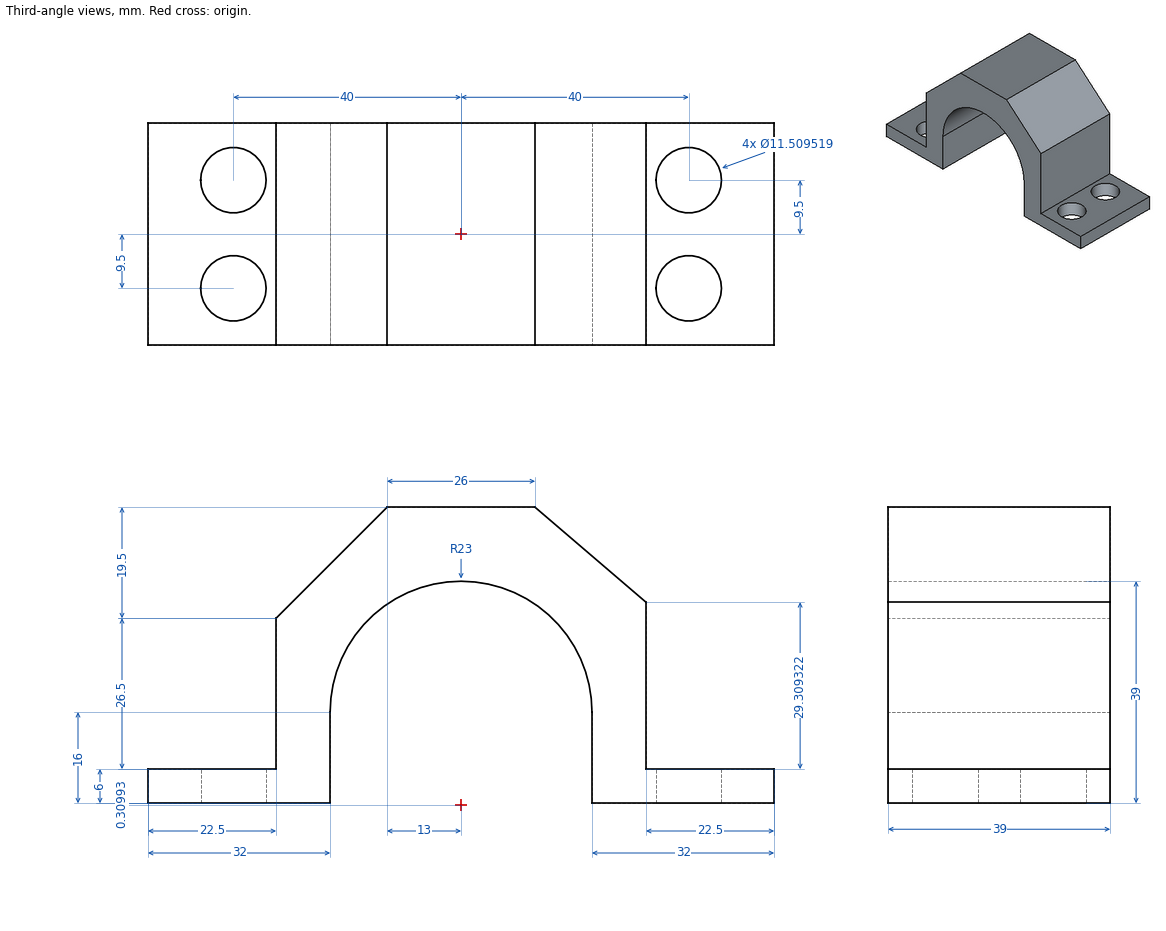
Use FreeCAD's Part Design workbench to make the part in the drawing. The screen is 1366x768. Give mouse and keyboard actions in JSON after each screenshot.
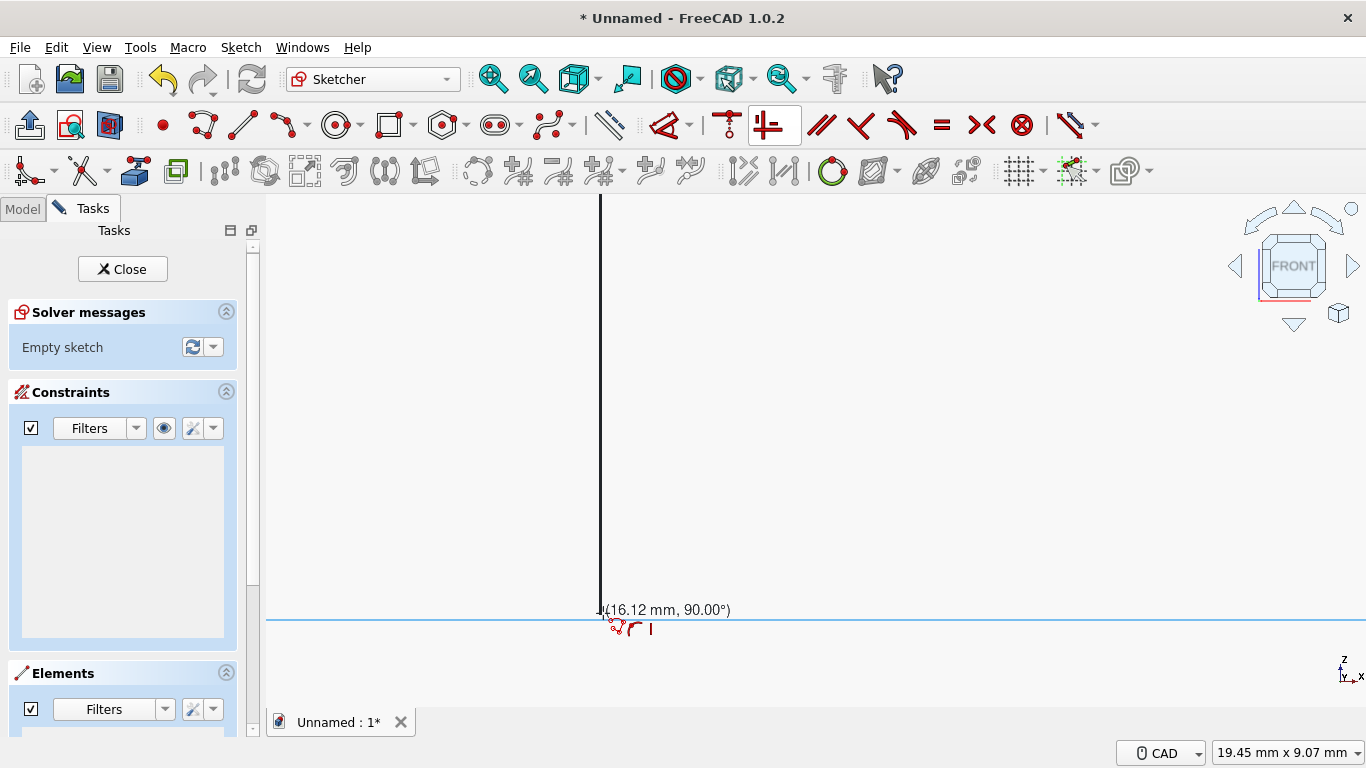
{"action": "left_click", "coordinate": [601, 603]}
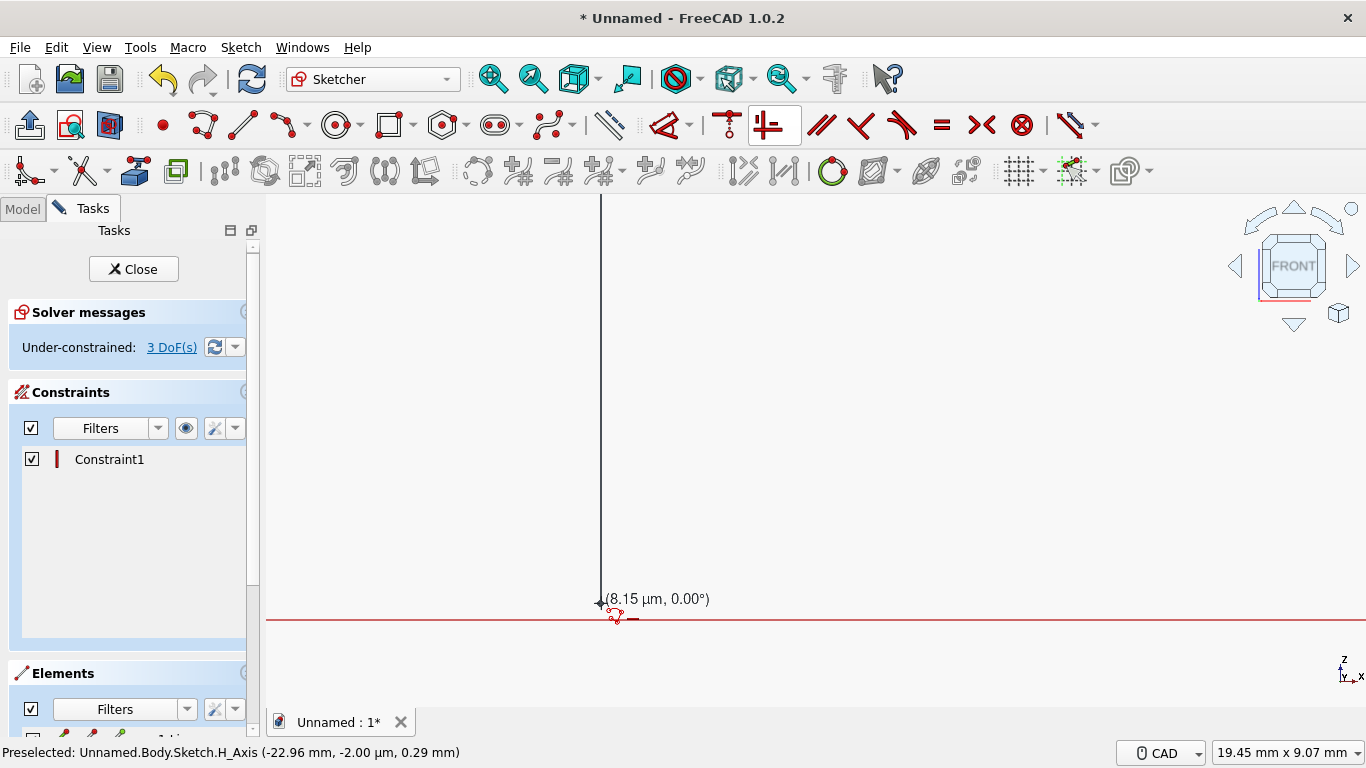
{"action": "scroll", "coordinate": [604, 614], "scroll_direction": "down", "scroll_amount": 11}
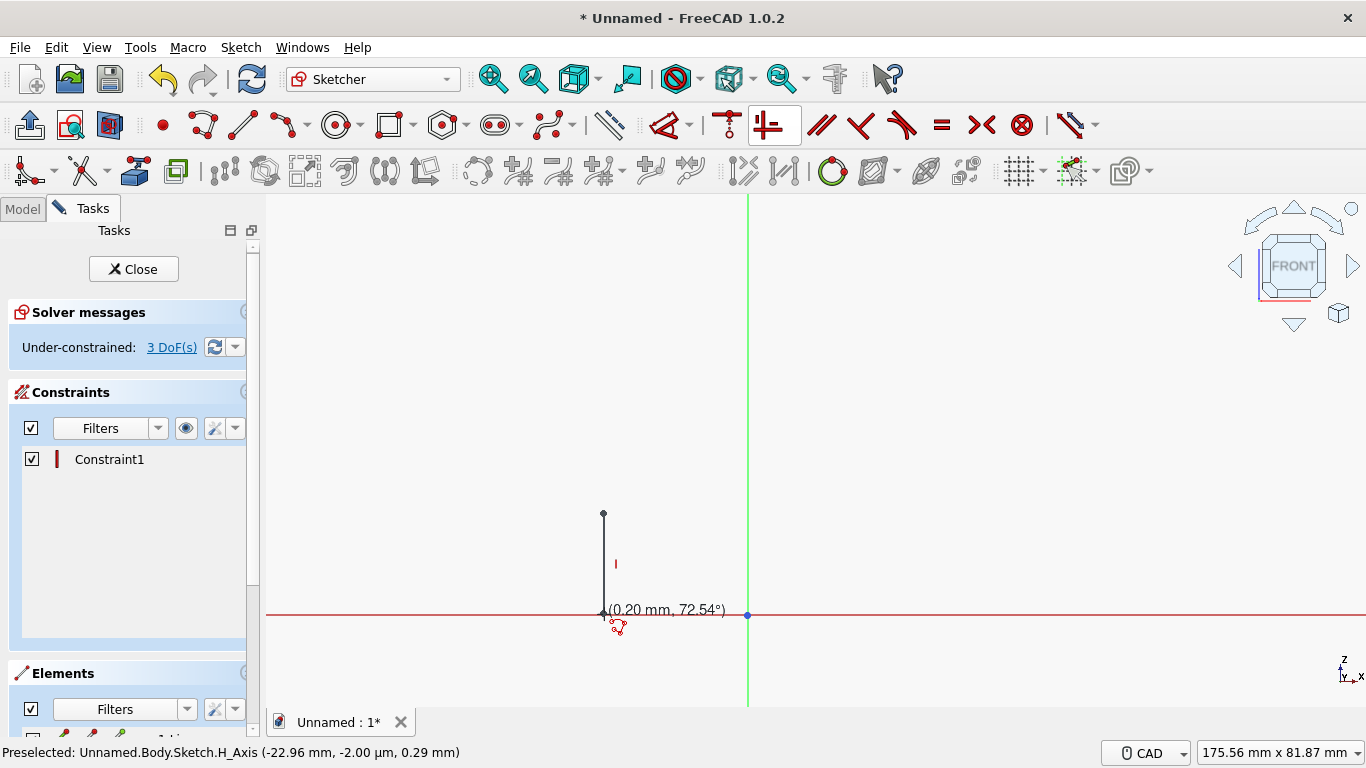
{"action": "scroll", "coordinate": [403, 614], "scroll_direction": "up", "scroll_amount": 11}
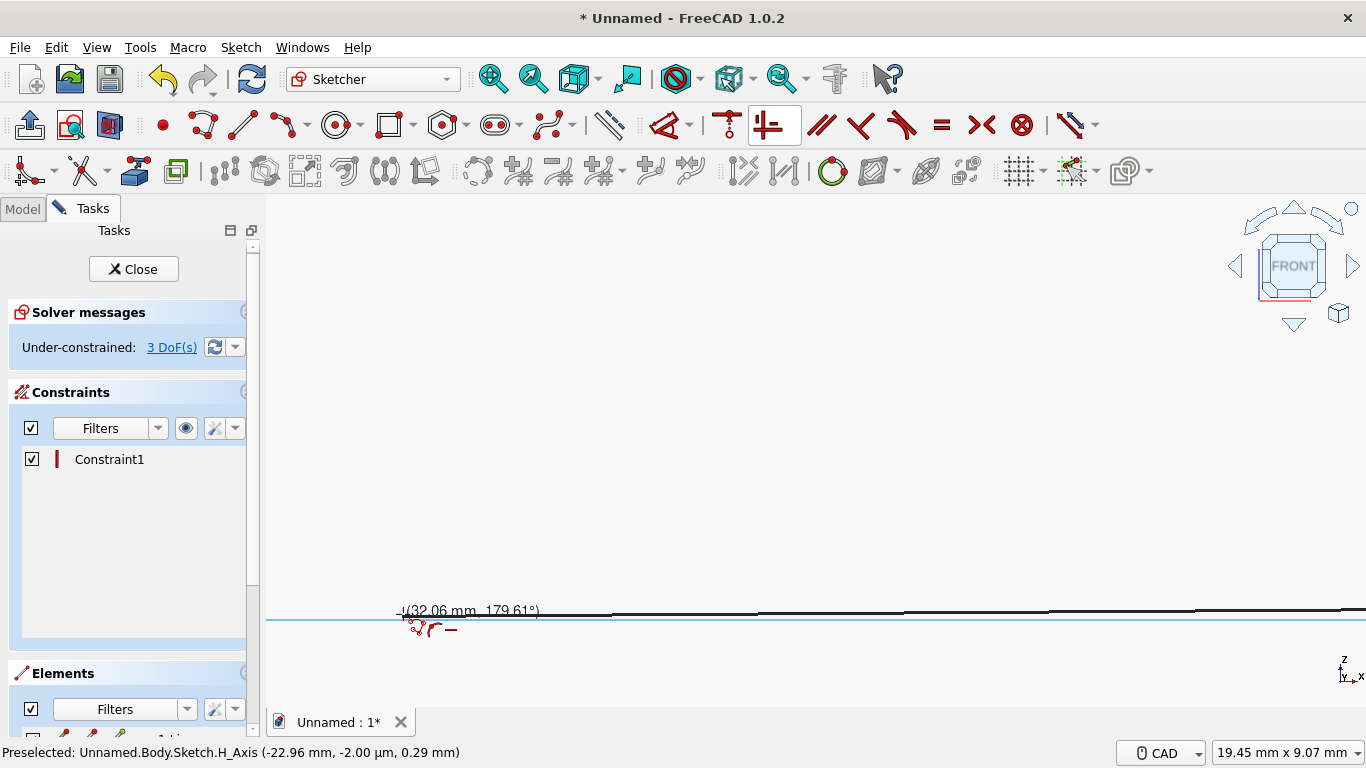
{"action": "left_click", "coordinate": [405, 603]}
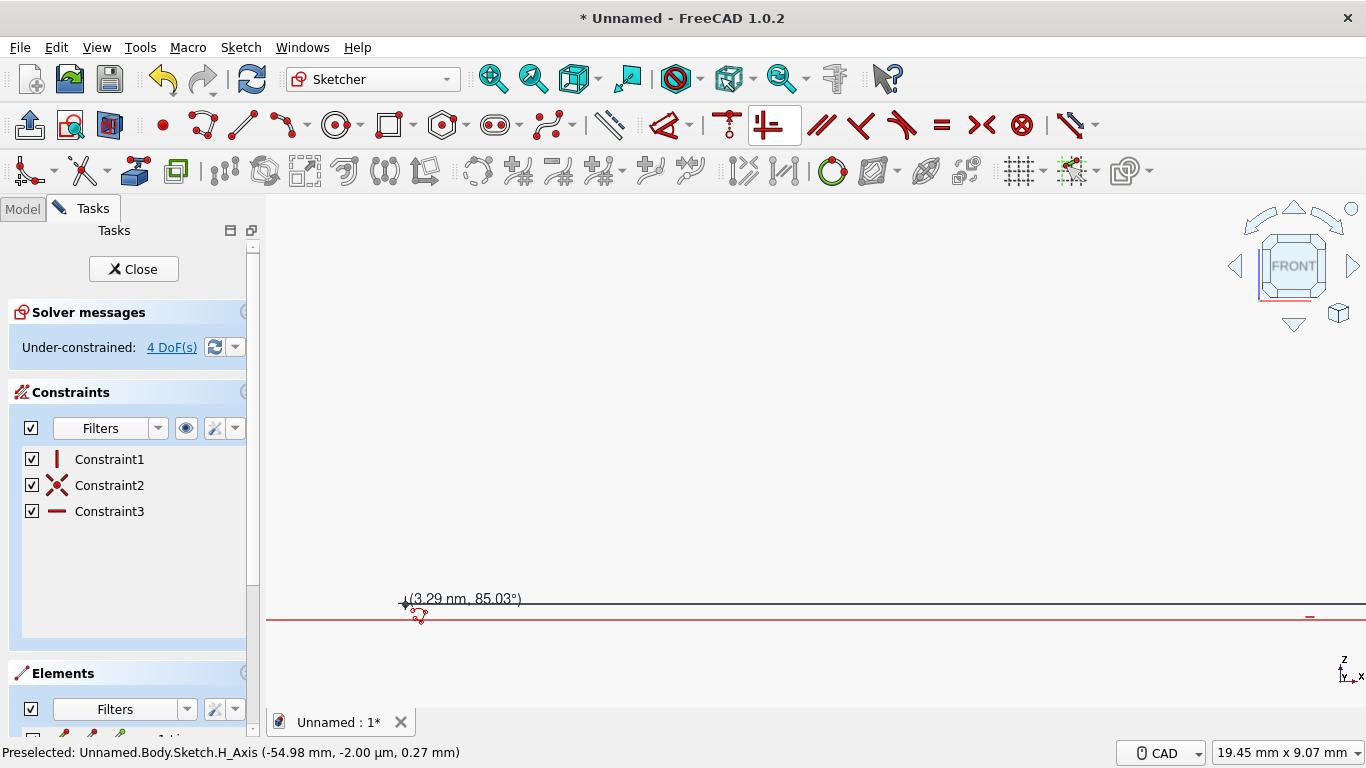
{"action": "scroll", "coordinate": [403, 614], "scroll_direction": "down", "scroll_amount": 11}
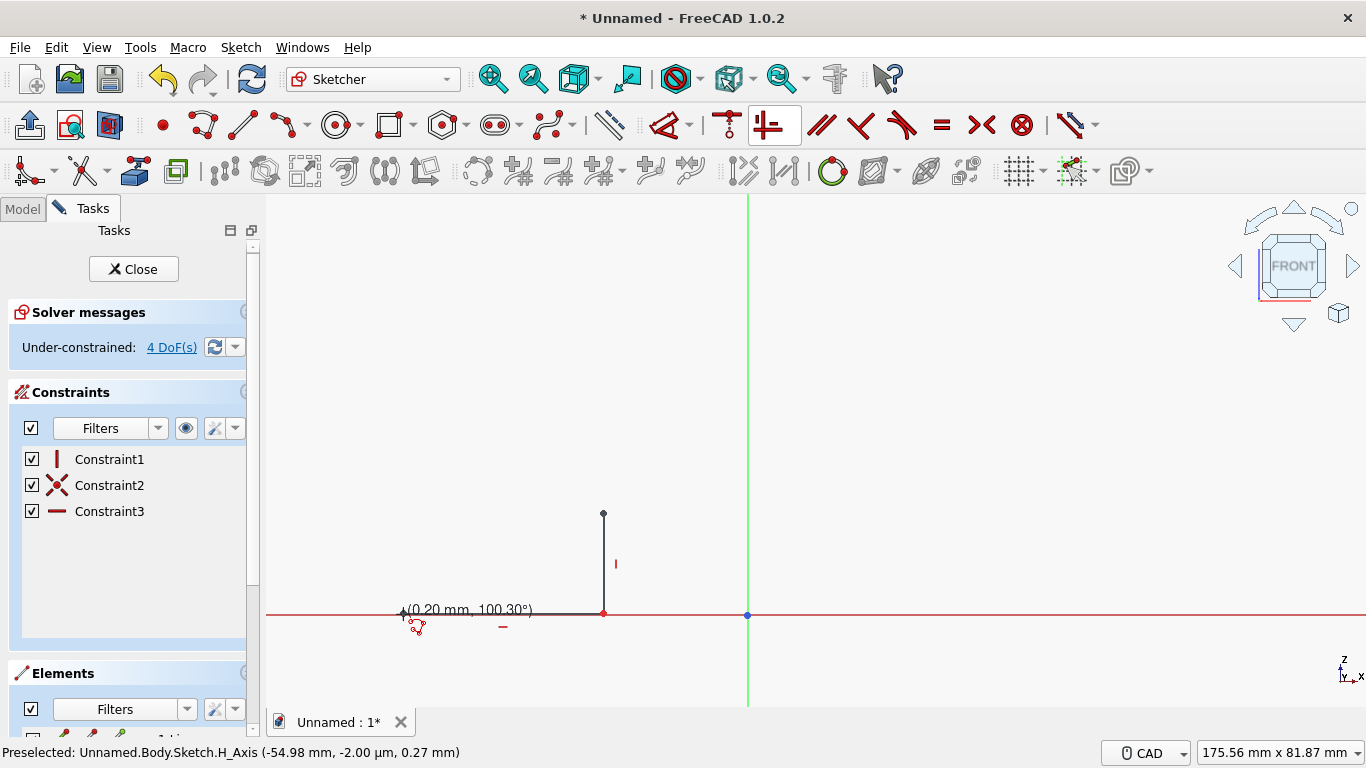
{"action": "left_click", "coordinate": [403, 576]}
{"action": "left_click", "coordinate": [544, 576]}
{"action": "left_click", "coordinate": [544, 410]}
{"action": "left_click", "coordinate": [666, 288]}
{"action": "left_click", "coordinate": [829, 288]}
{"action": "left_click", "coordinate": [952, 392]}
{"action": "left_click", "coordinate": [952, 576]}
{"action": "left_click", "coordinate": [1093, 576]}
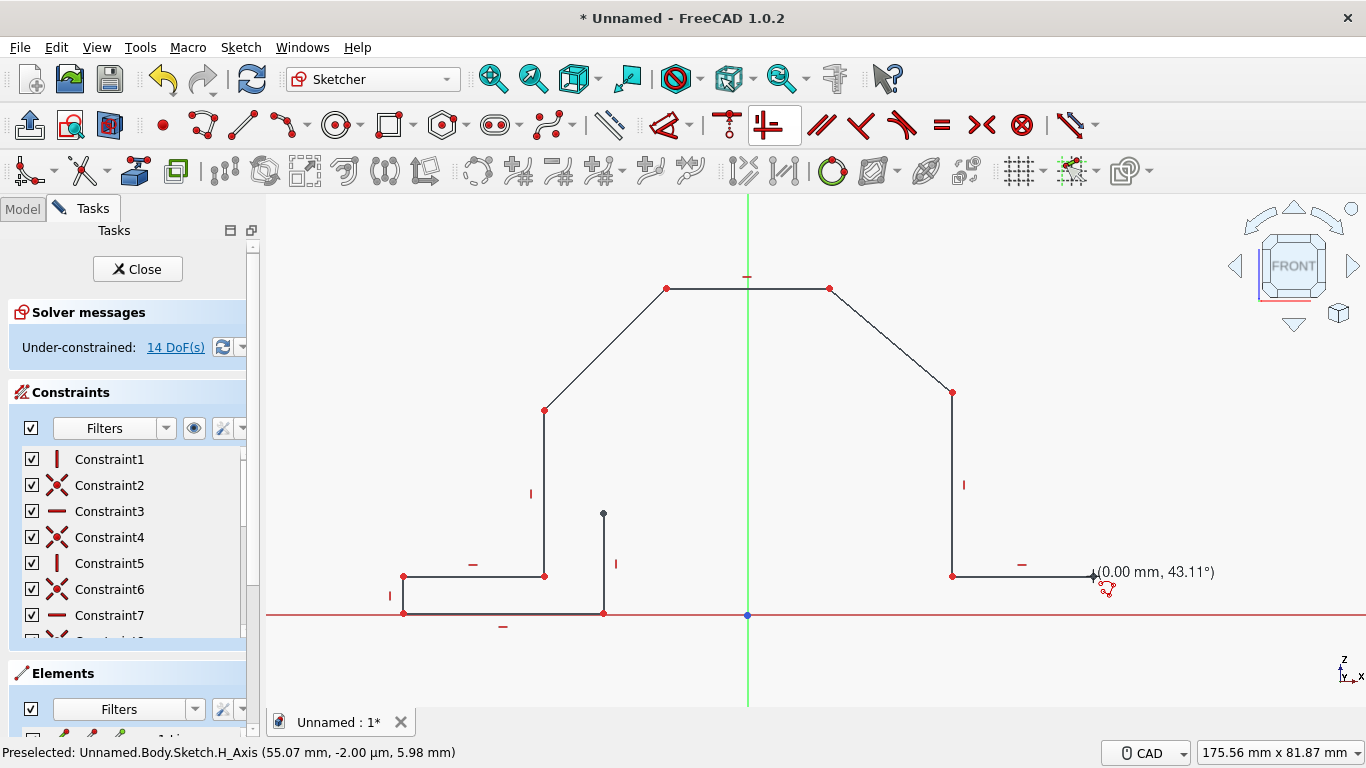
{"action": "scroll", "coordinate": [1093, 614], "scroll_direction": "up", "scroll_amount": 11}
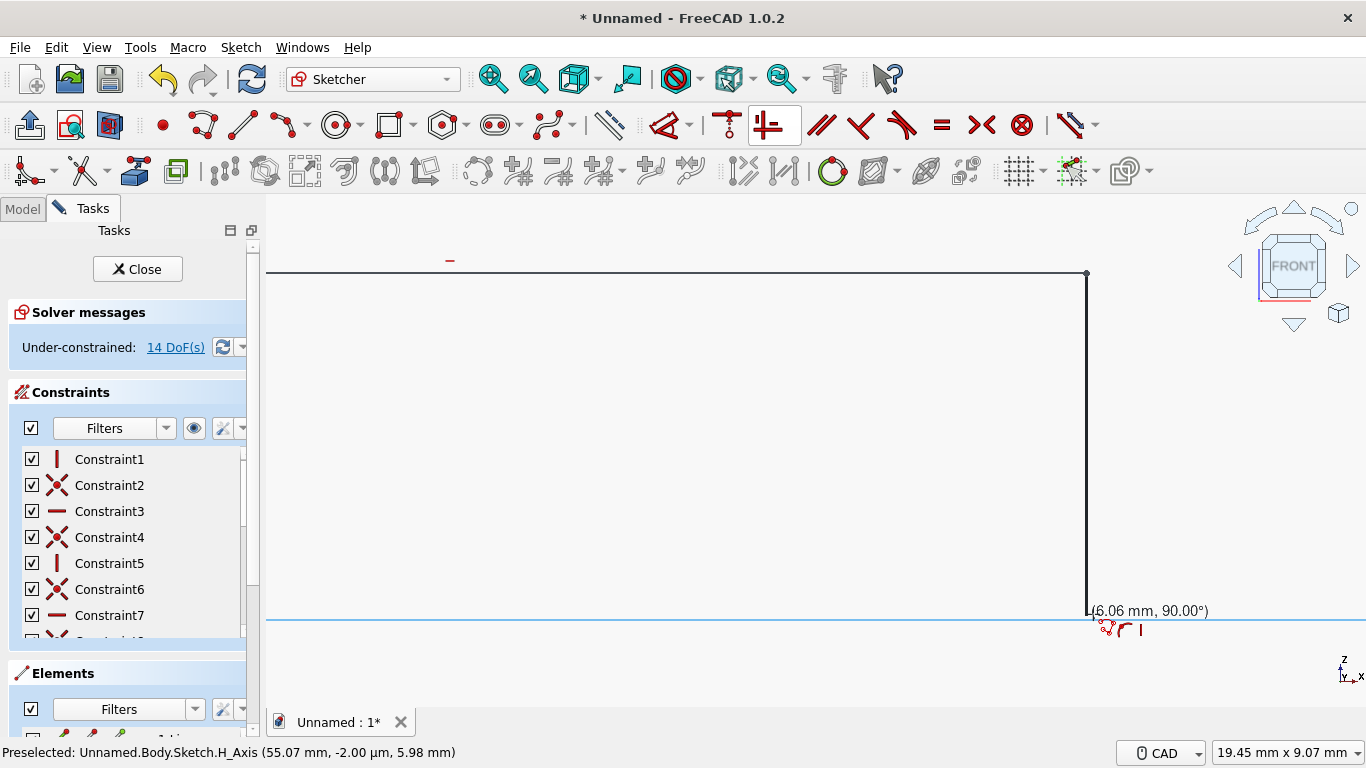
{"action": "left_click", "coordinate": [1087, 603]}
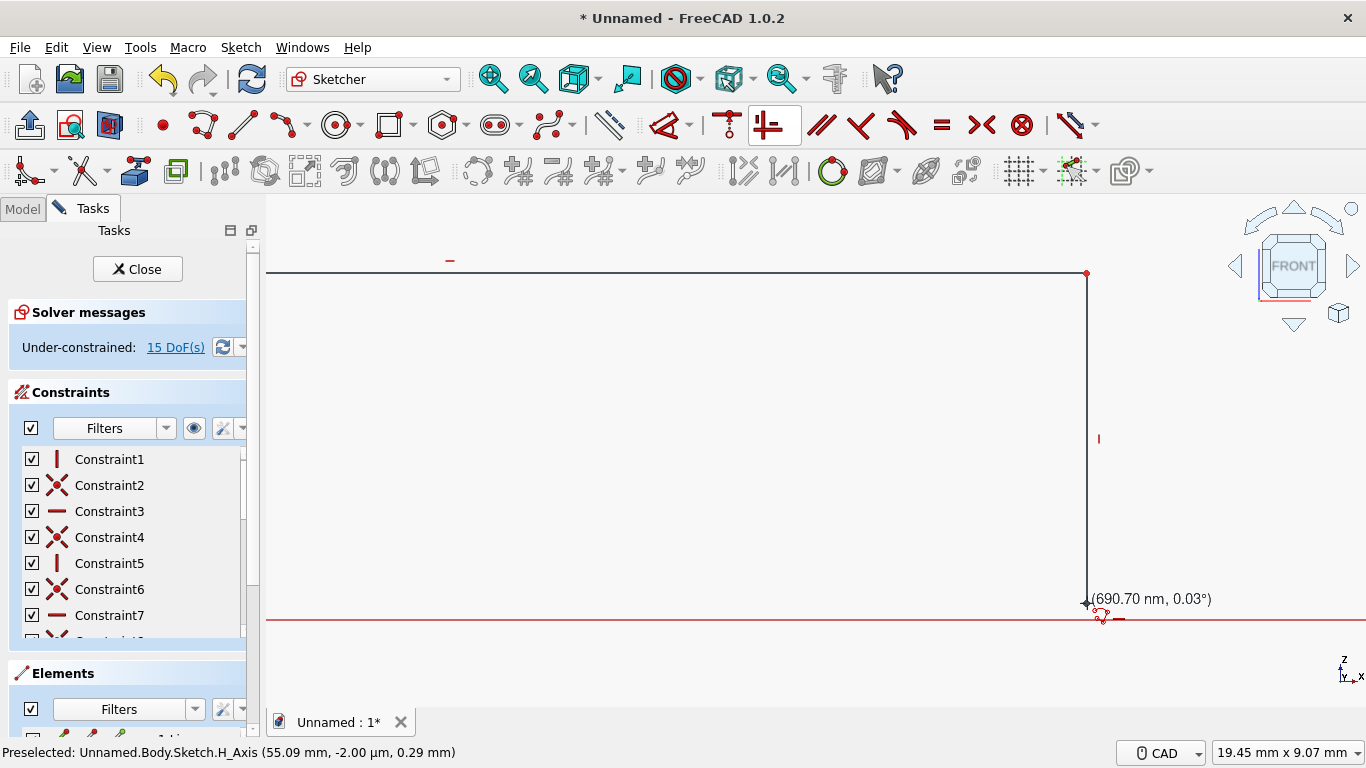
{"action": "scroll", "coordinate": [1093, 614], "scroll_direction": "down", "scroll_amount": 11}